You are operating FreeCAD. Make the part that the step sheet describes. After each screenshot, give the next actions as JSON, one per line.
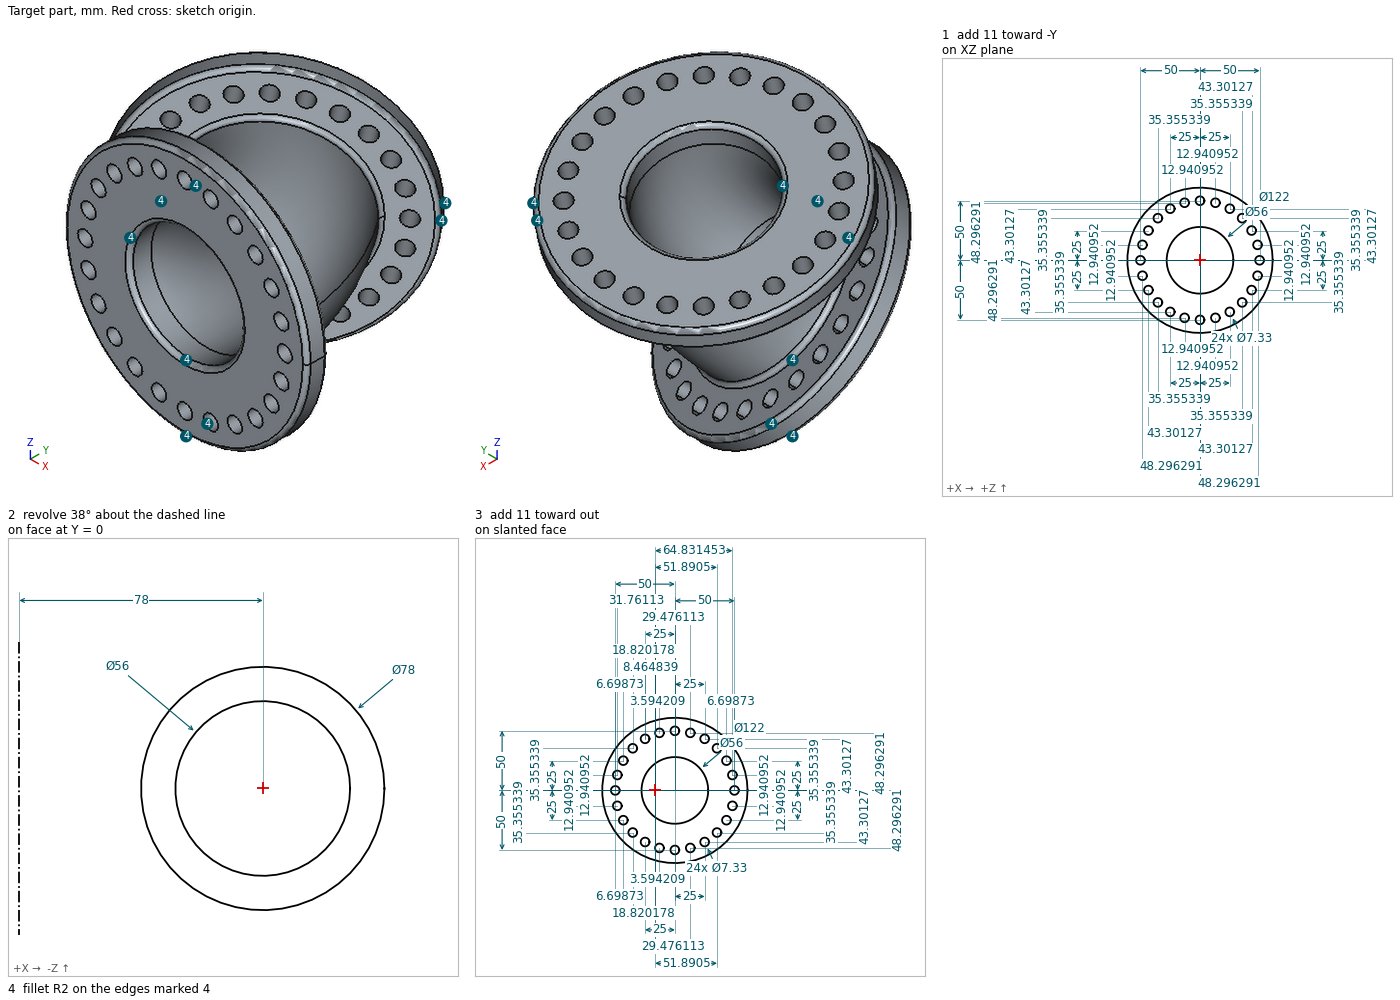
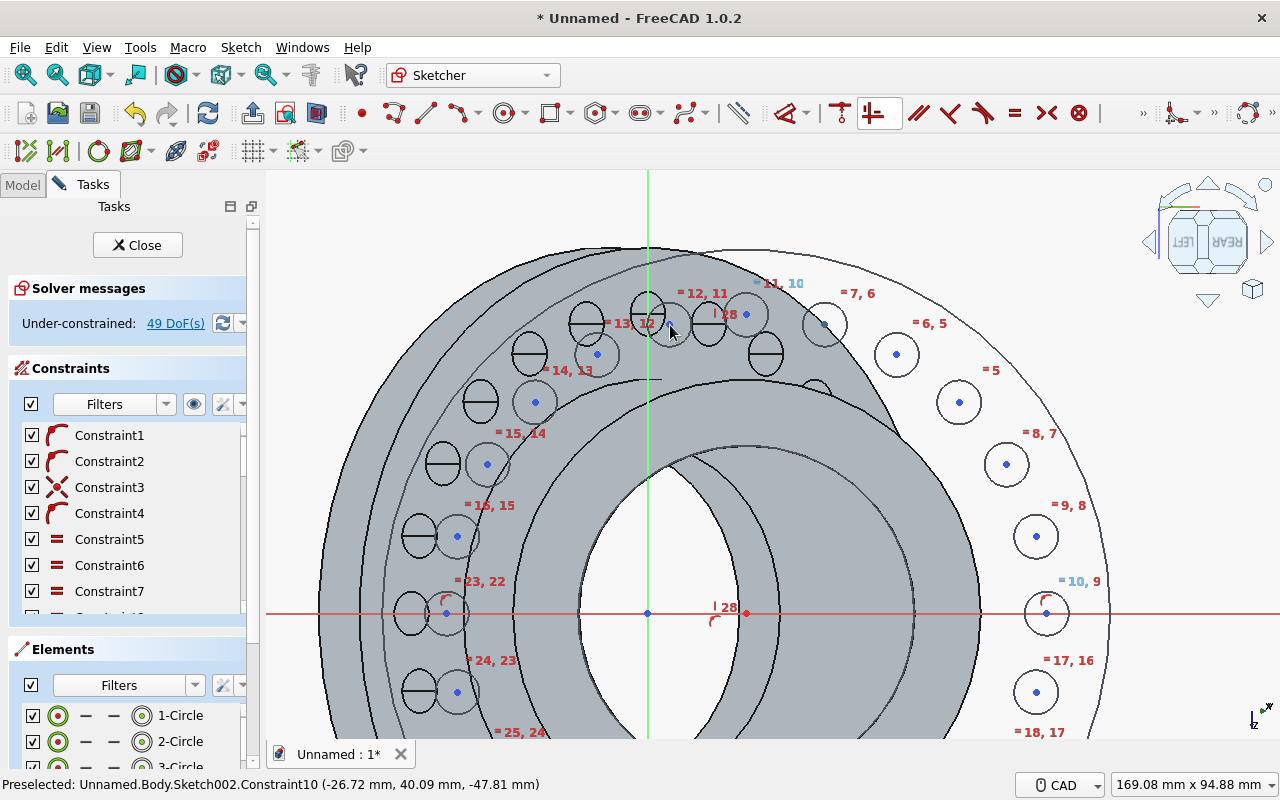
{"action": "left_click", "coordinate": [669, 325]}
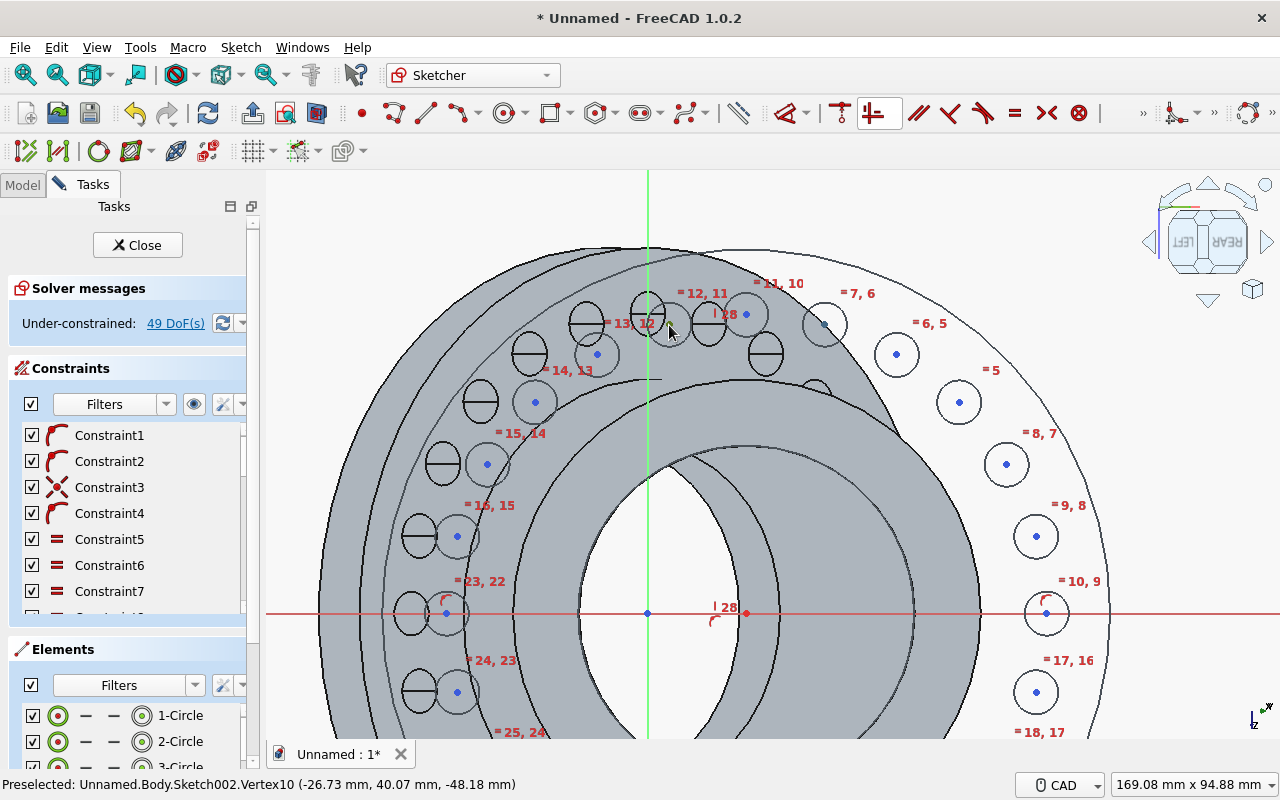
{"action": "left_click", "coordinate": [896, 114]}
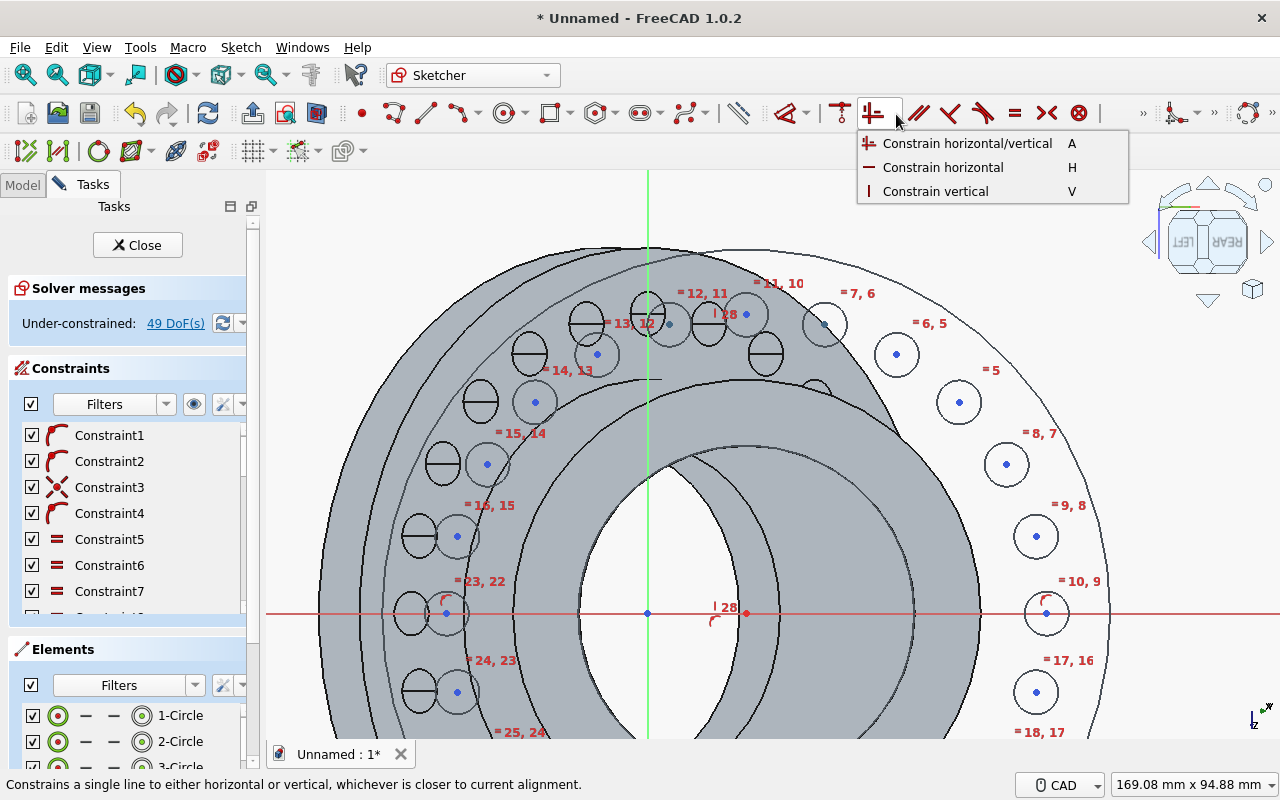
{"action": "left_click", "coordinate": [993, 167]}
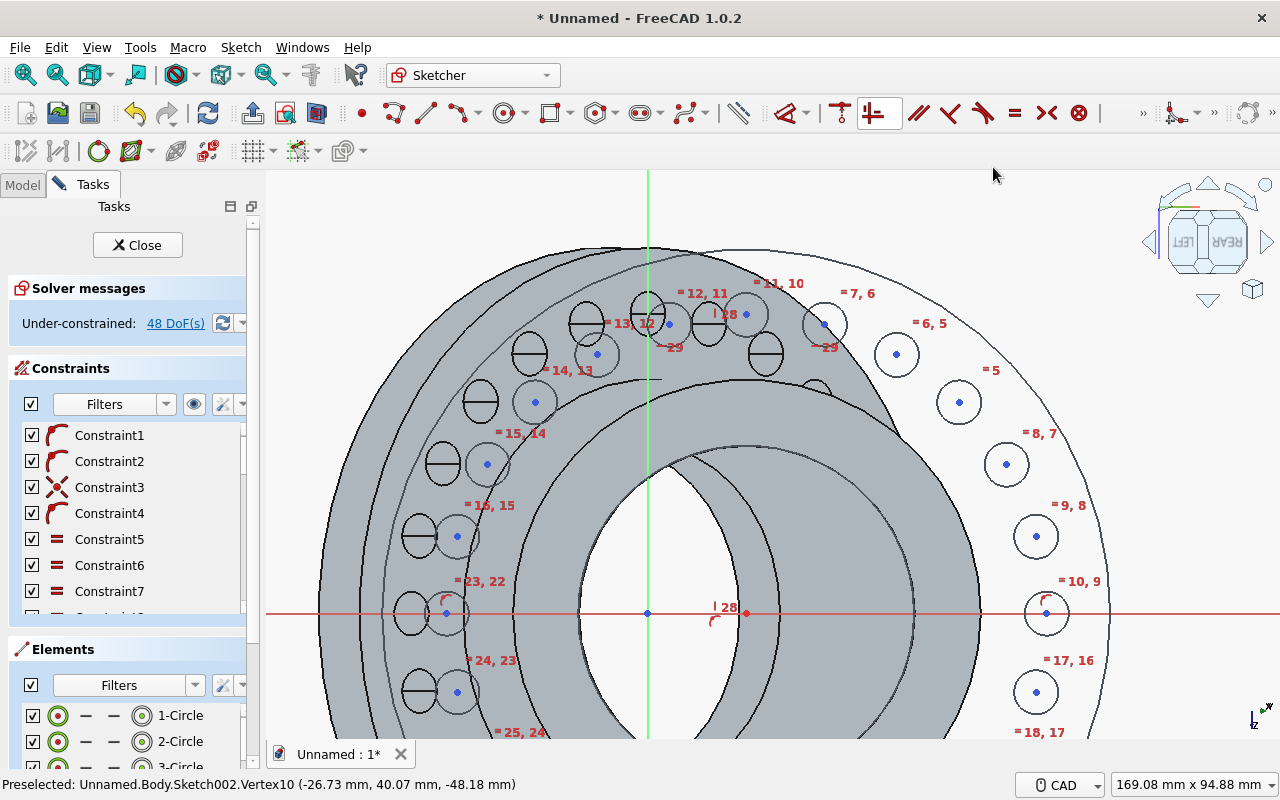
{"action": "left_click", "coordinate": [897, 355]}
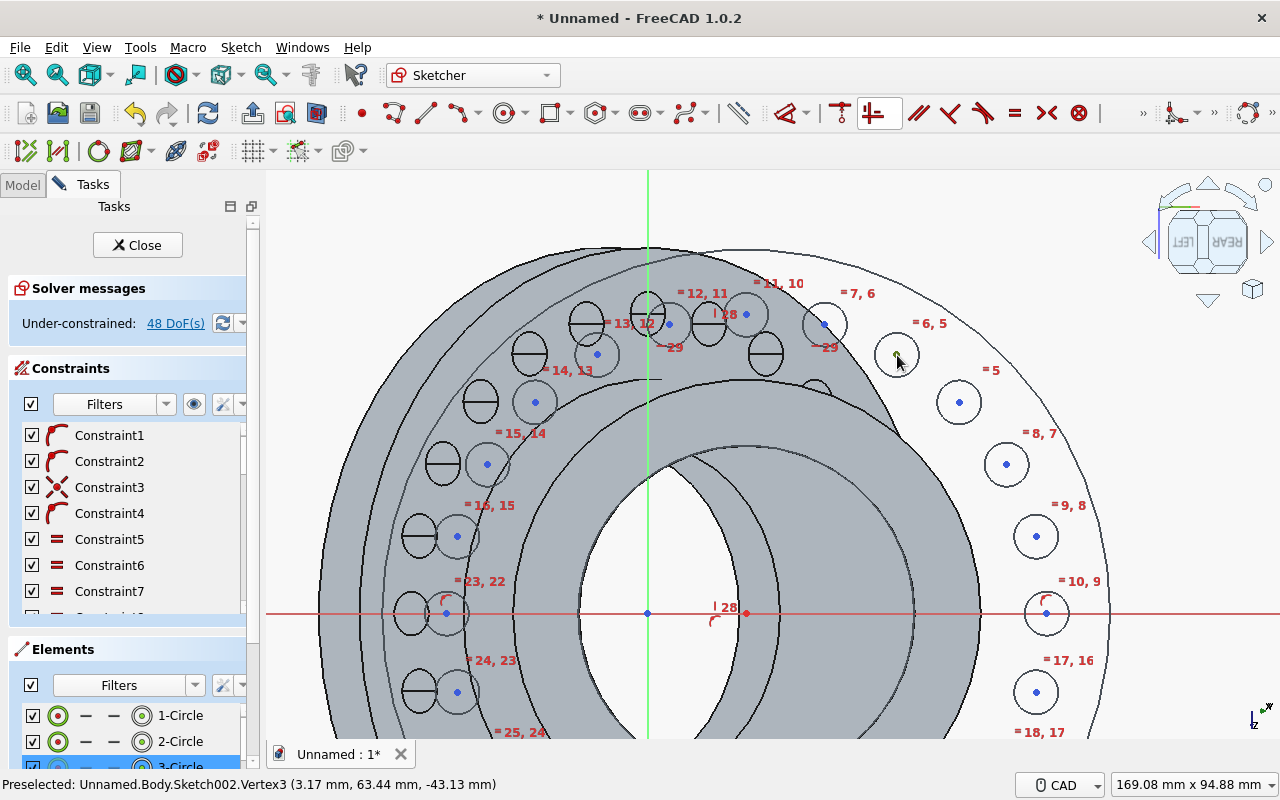
{"action": "left_click", "coordinate": [597, 355]}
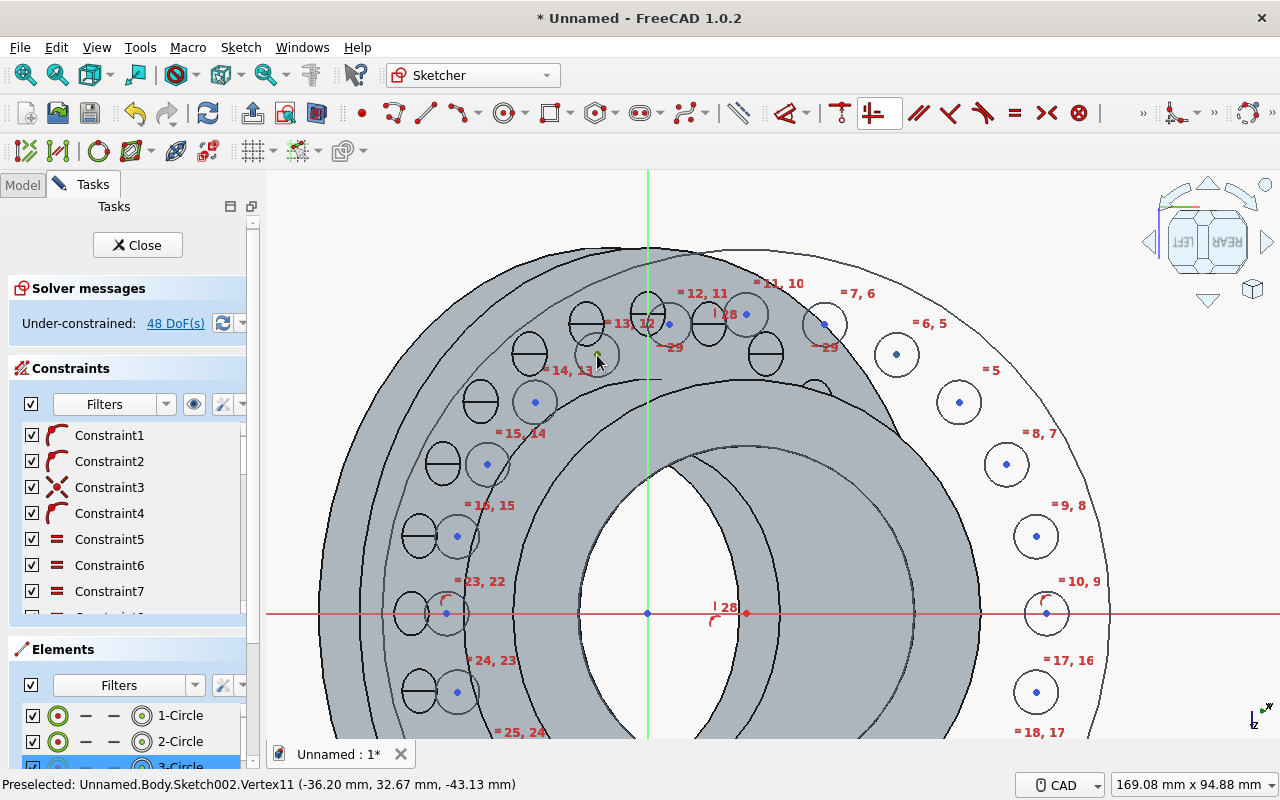
{"action": "key", "text": "h"}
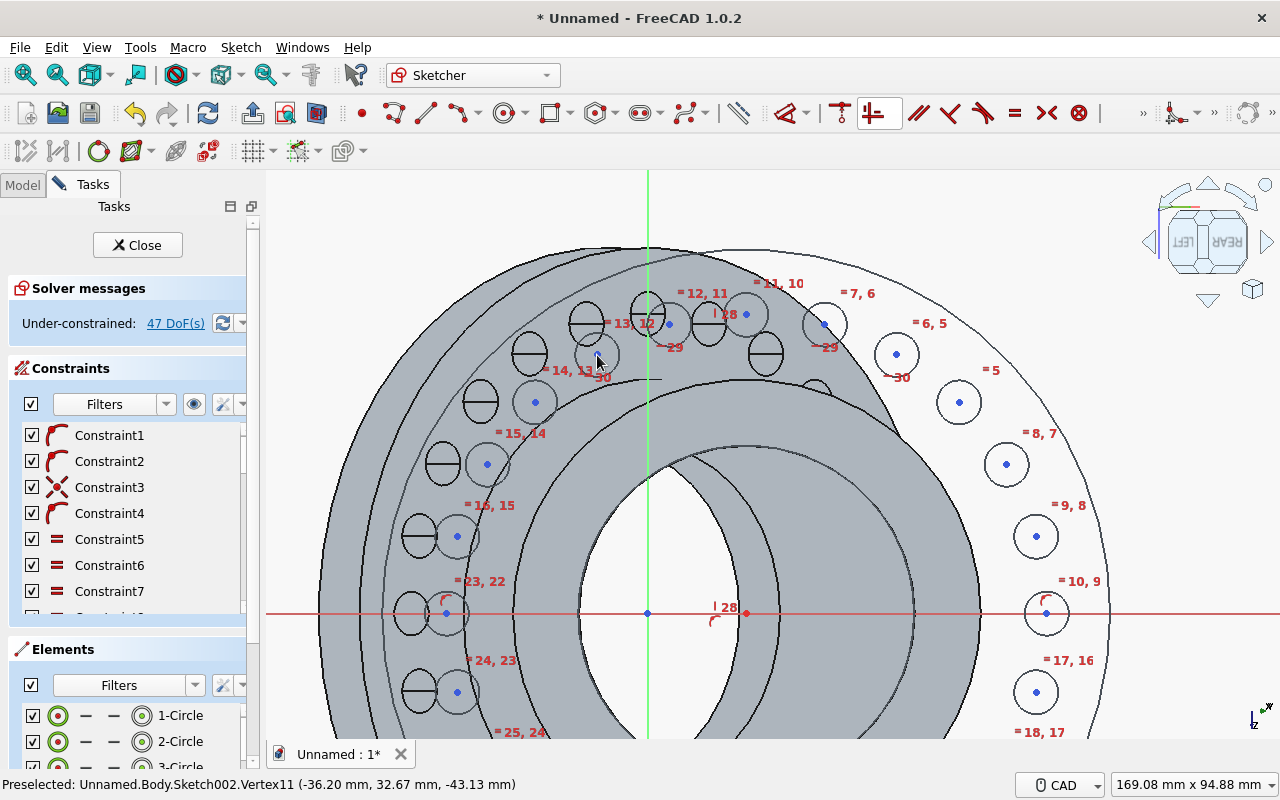
{"action": "left_click", "coordinate": [1036, 537]}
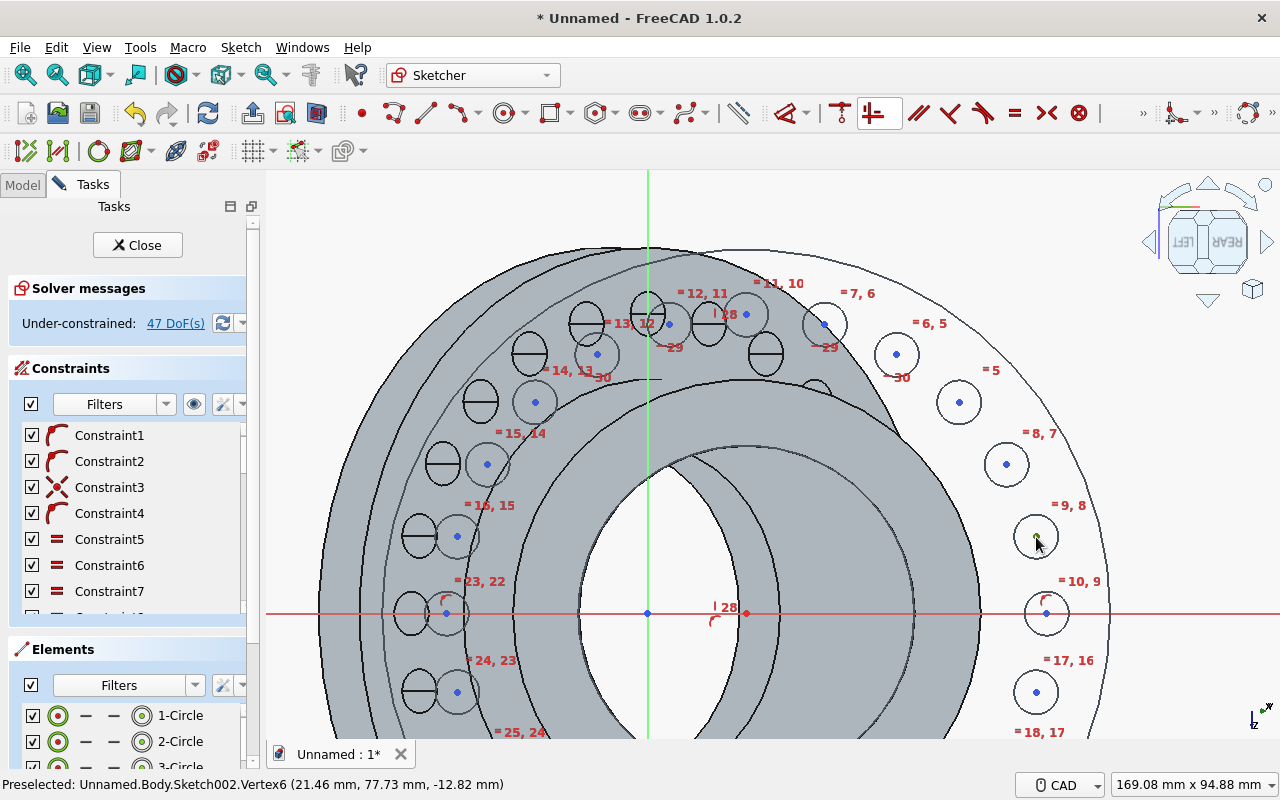
{"action": "left_click", "coordinate": [1036, 692]}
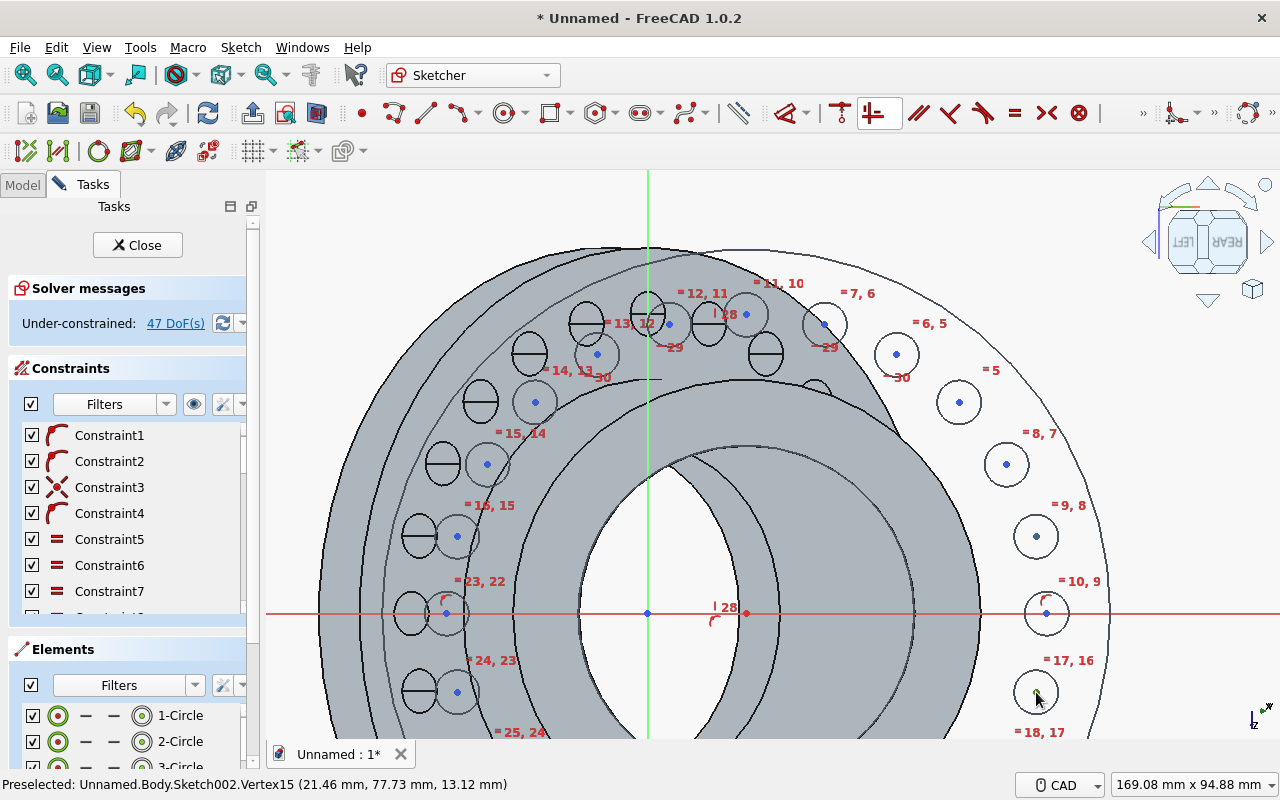
{"action": "left_click", "coordinate": [896, 114]}